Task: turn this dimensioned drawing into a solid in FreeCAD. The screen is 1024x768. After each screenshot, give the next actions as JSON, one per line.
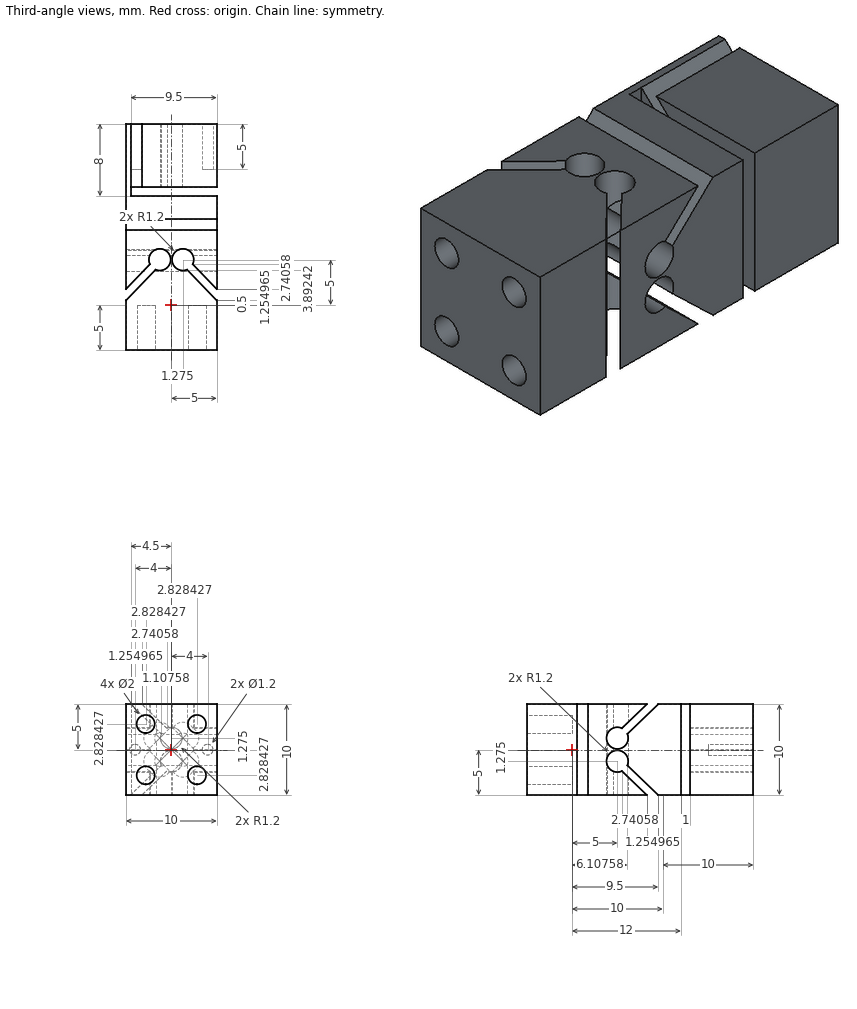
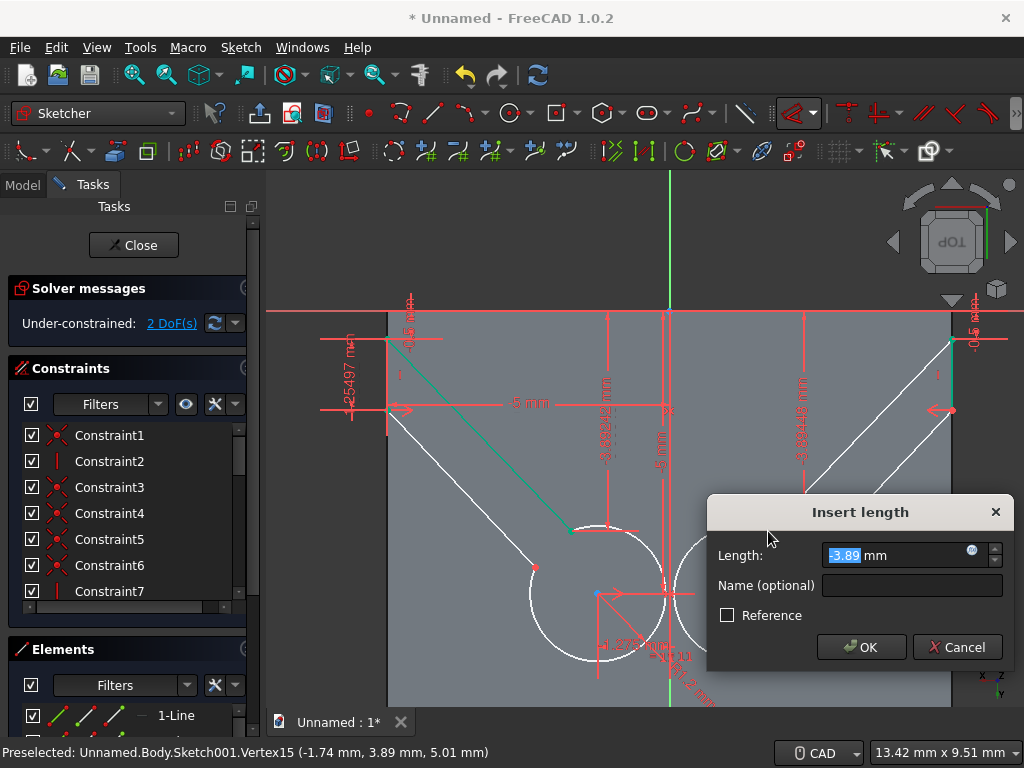
{"action": "type", "text": "-3.89242"}
{"action": "key", "text": "Return"}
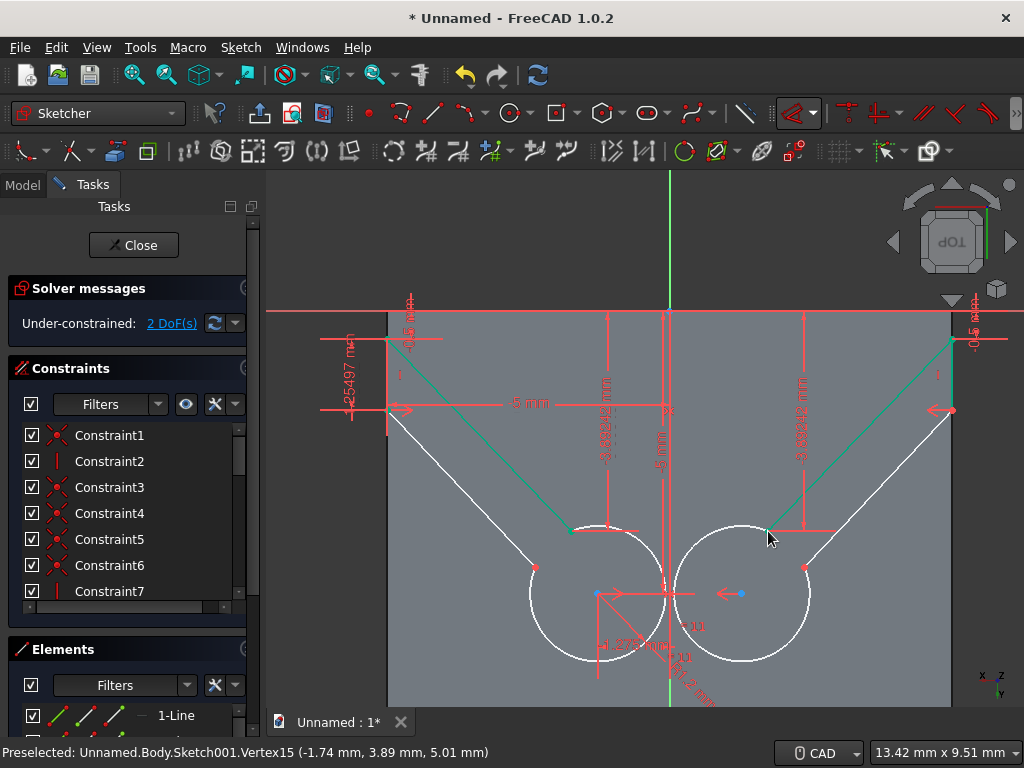
{"action": "left_click", "coordinate": [432, 457]}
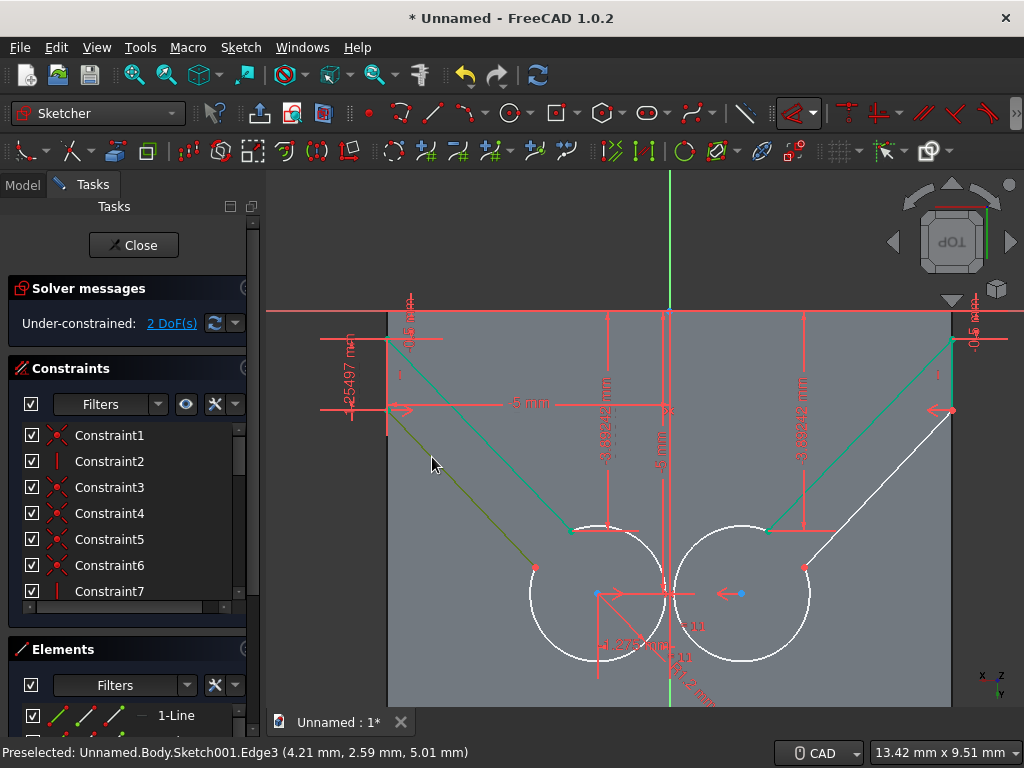
{"action": "left_click", "coordinate": [816, 114]}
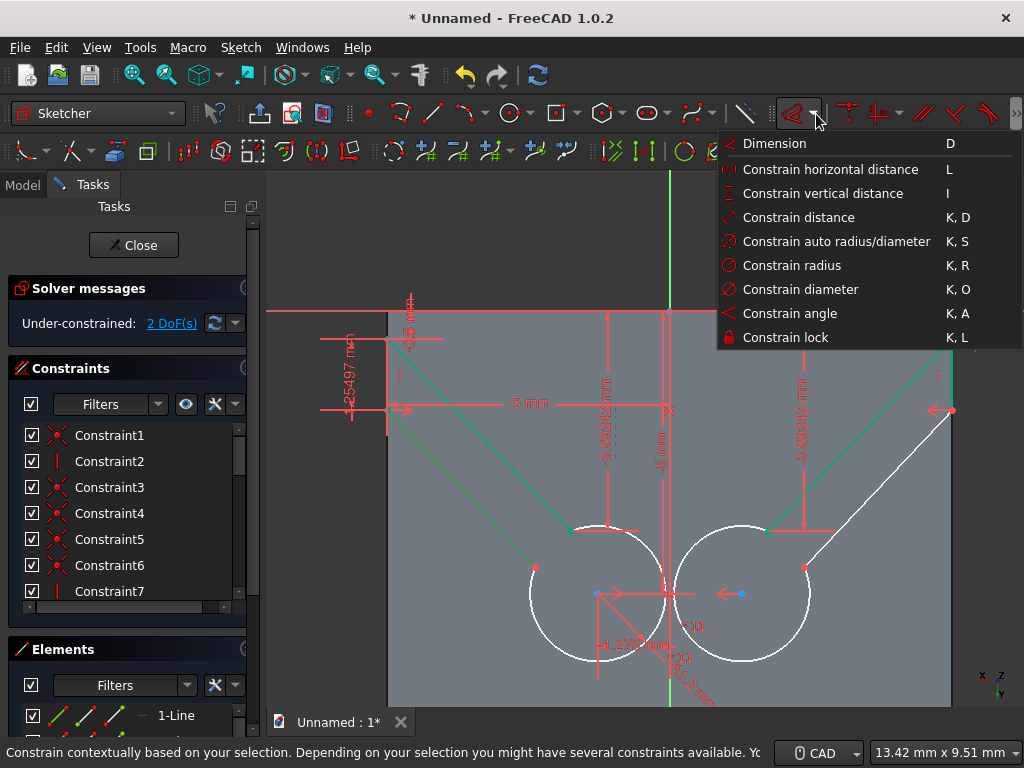
{"action": "left_click", "coordinate": [870, 193]}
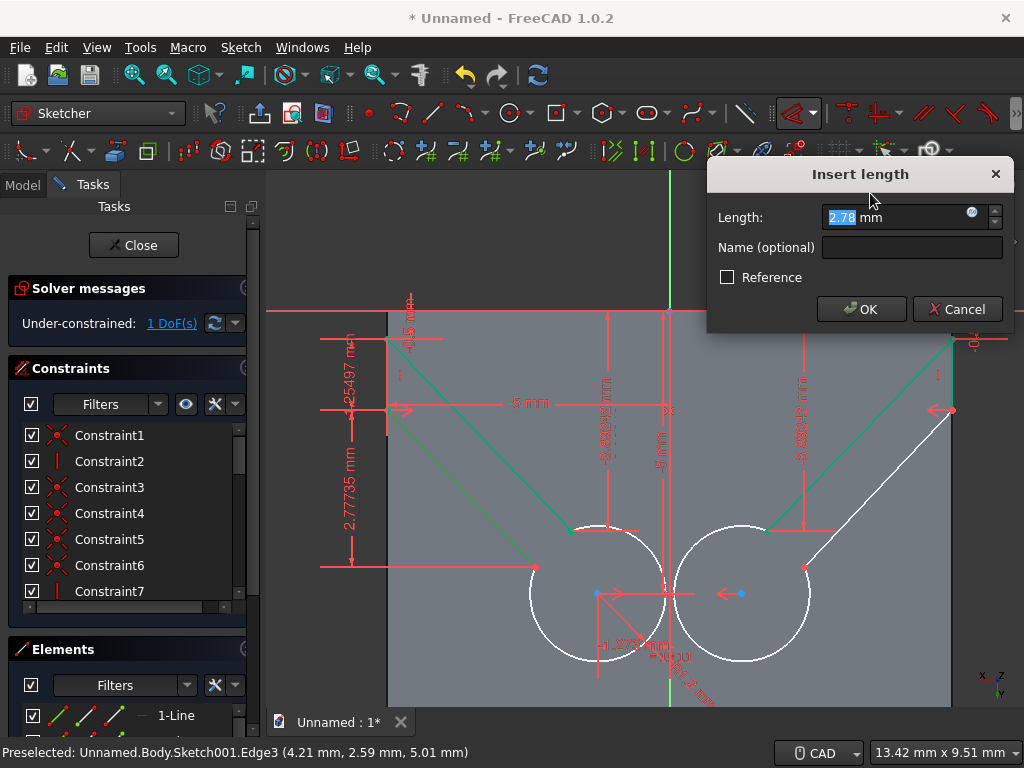
{"action": "type", "text": "2.74058"}
{"action": "key", "text": "Return"}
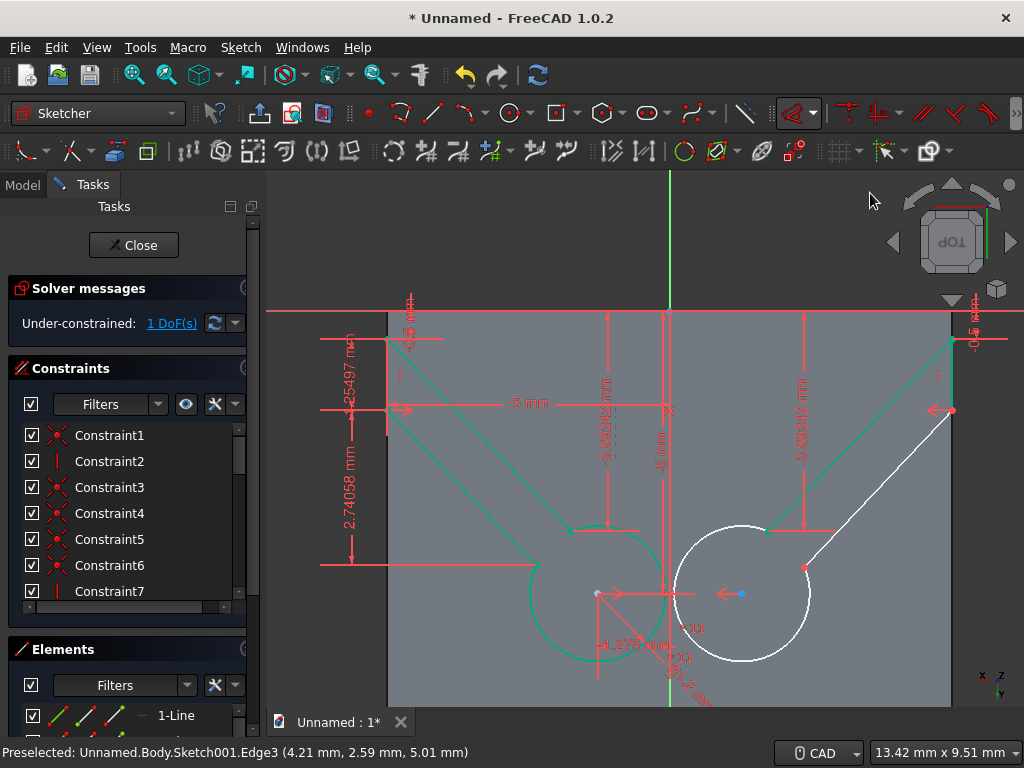
{"action": "left_click", "coordinate": [849, 520]}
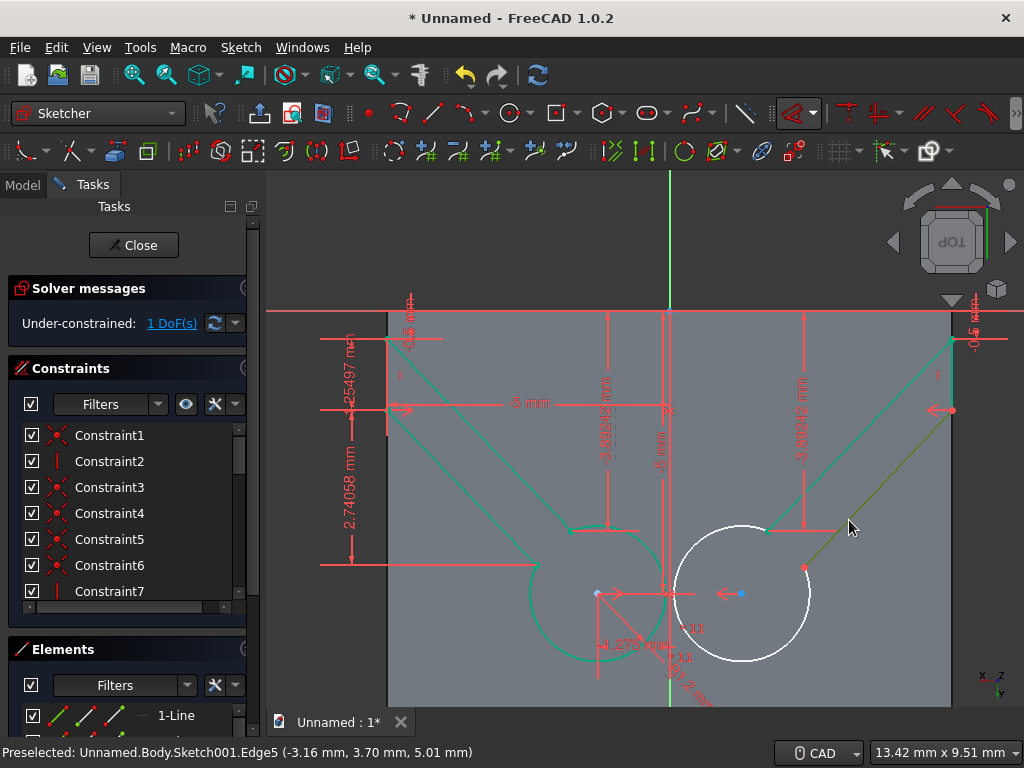
{"action": "left_click", "coordinate": [816, 114]}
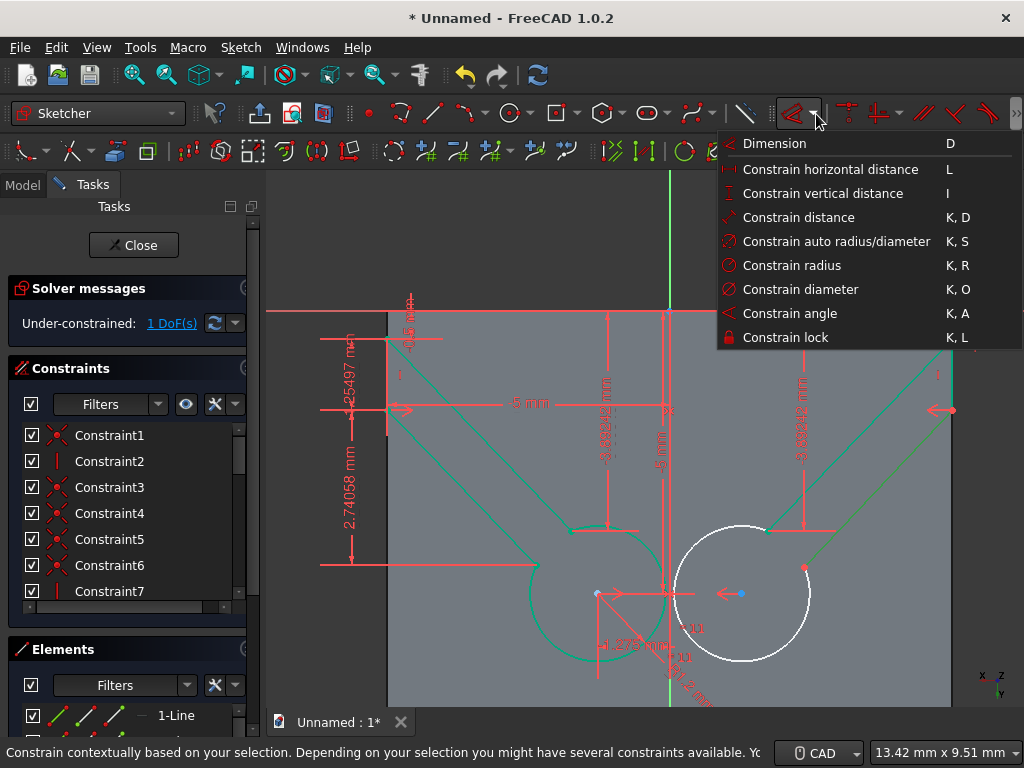
{"action": "left_click", "coordinate": [870, 193]}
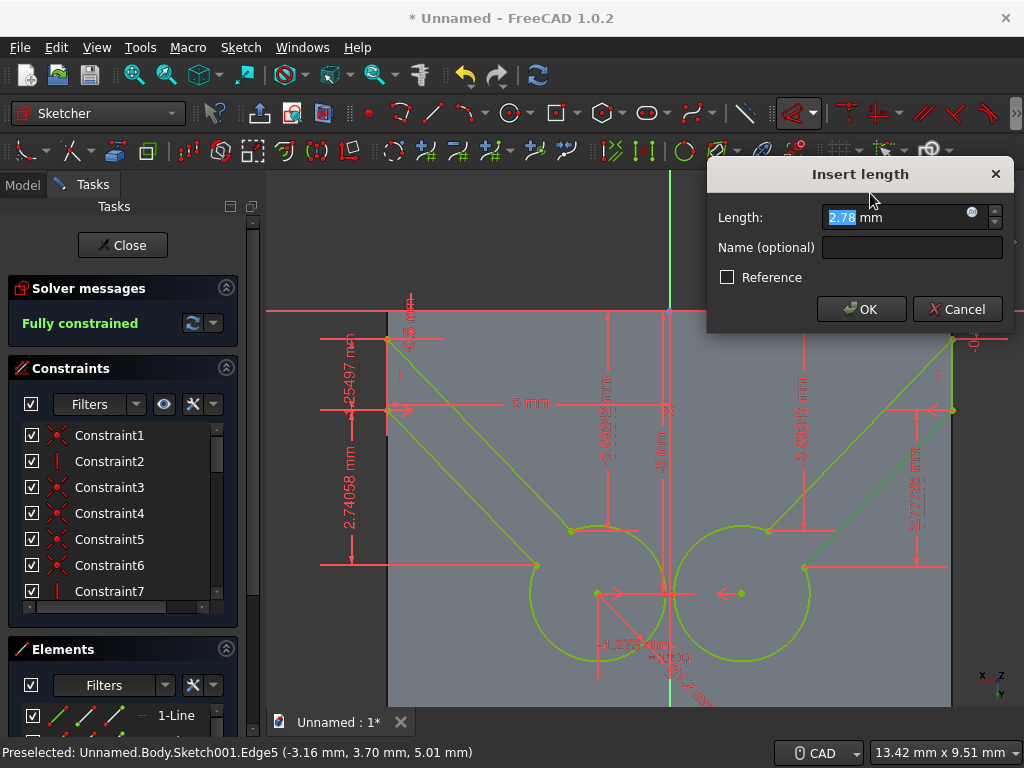
{"action": "type", "text": "2.74058"}
{"action": "key", "text": "Return"}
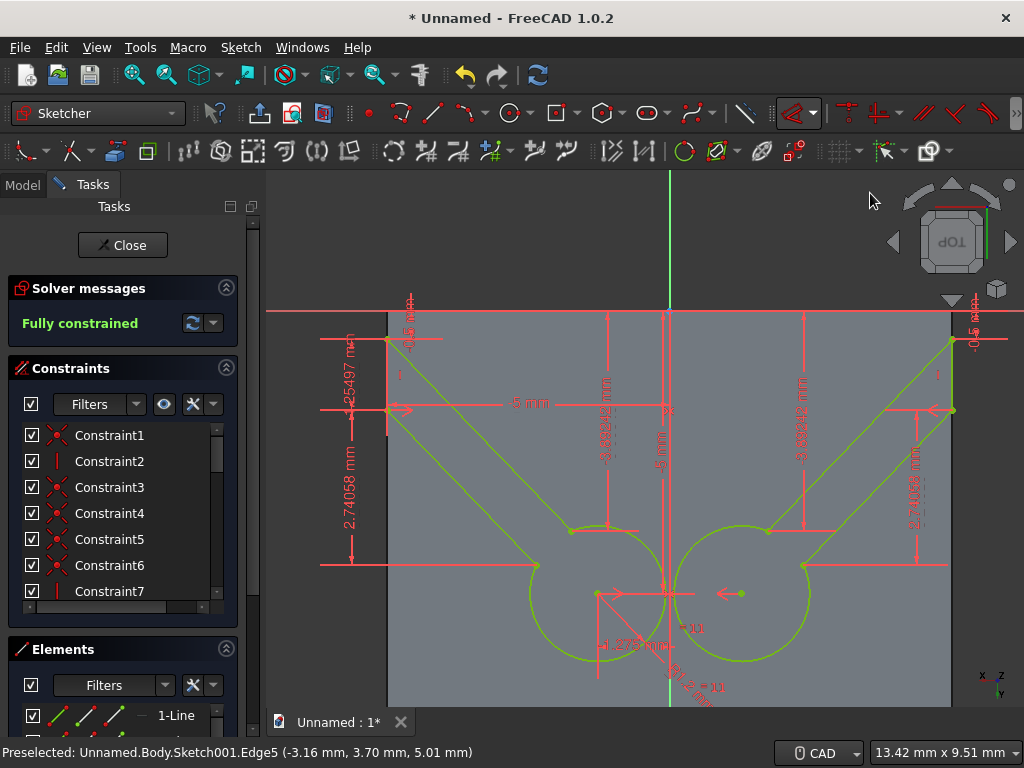
{"action": "left_click", "coordinate": [123, 245]}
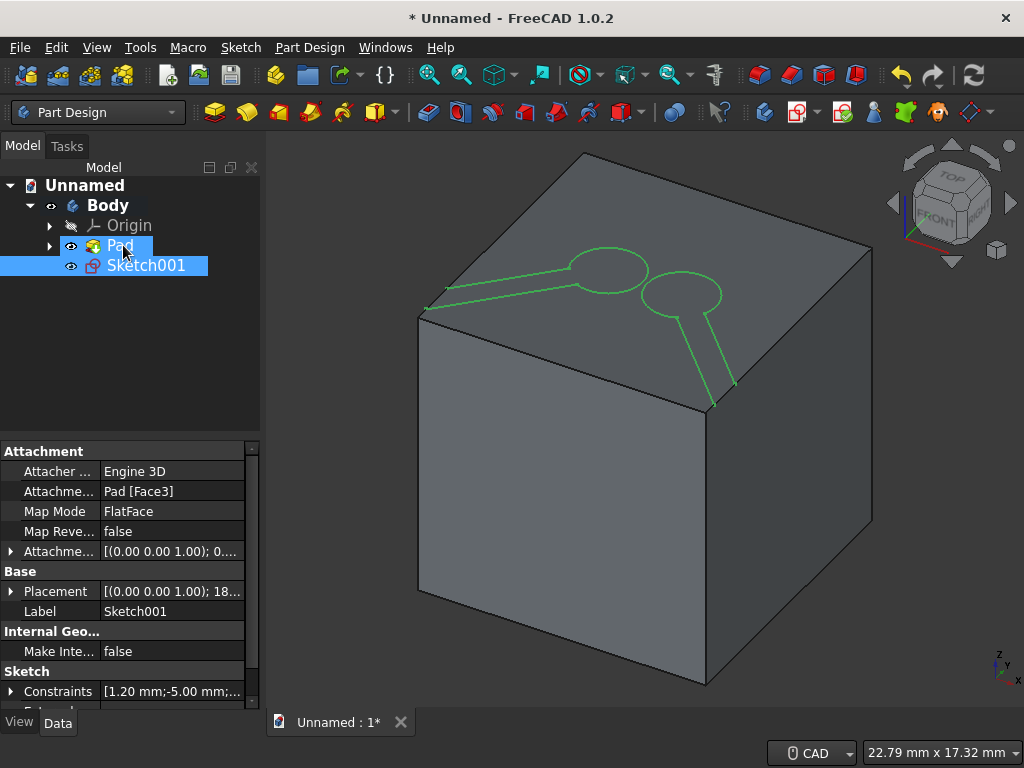
{"action": "left_click", "coordinate": [430, 112]}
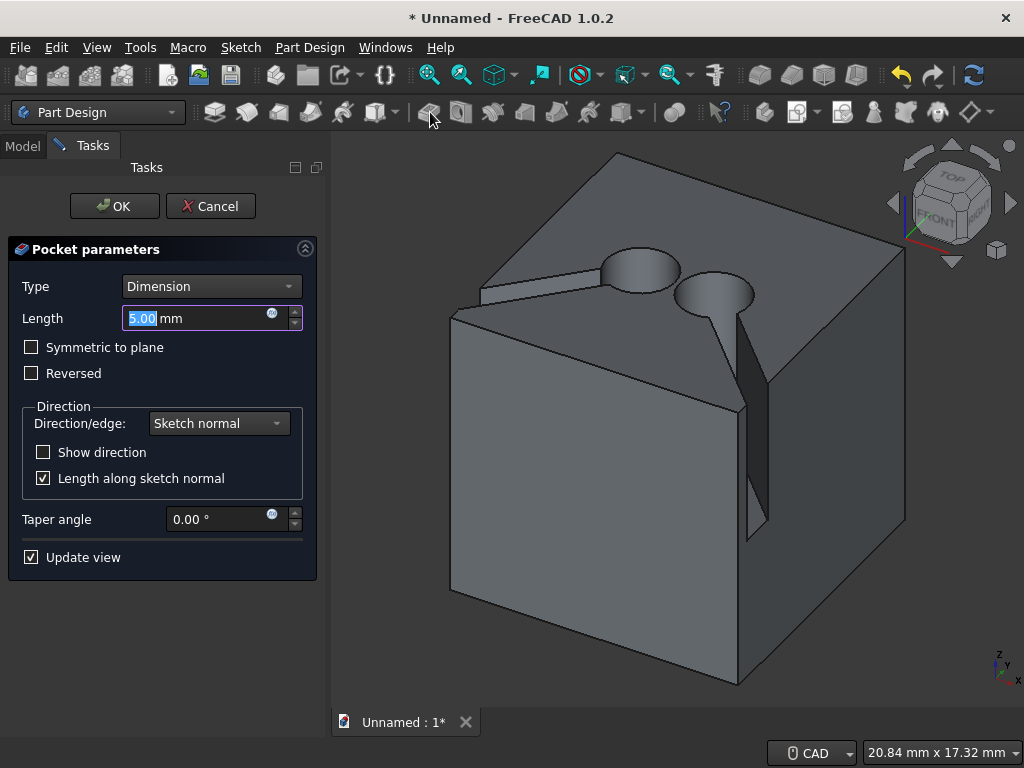
{"action": "left_click", "coordinate": [212, 286]}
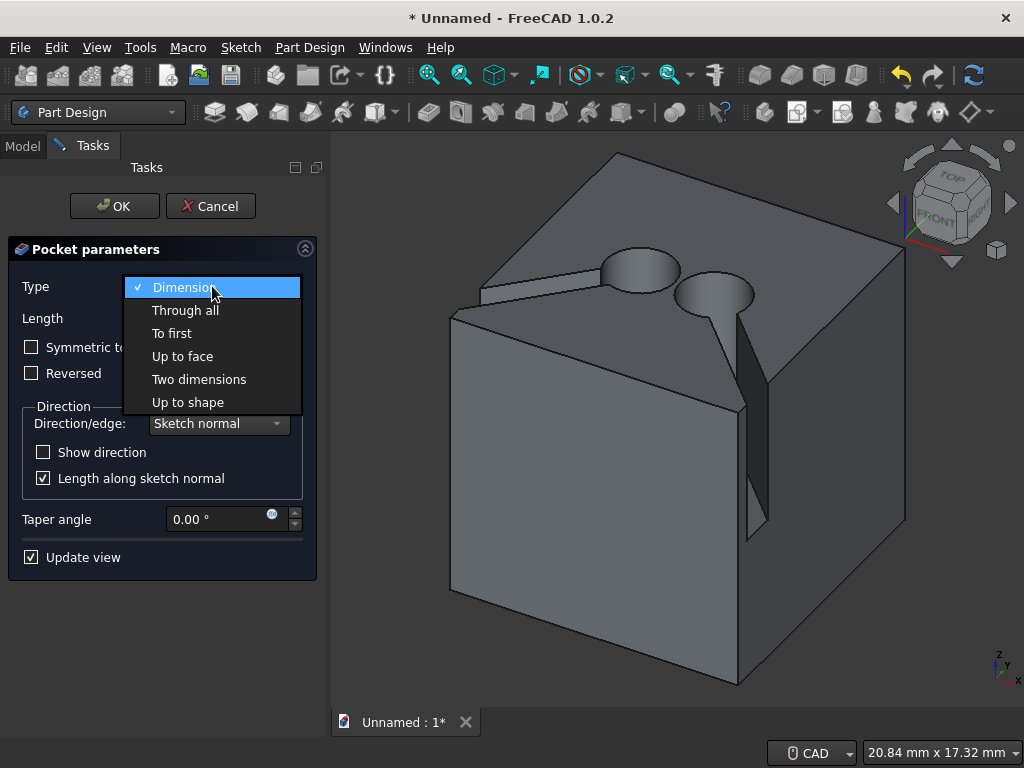
{"action": "left_click", "coordinate": [212, 310]}